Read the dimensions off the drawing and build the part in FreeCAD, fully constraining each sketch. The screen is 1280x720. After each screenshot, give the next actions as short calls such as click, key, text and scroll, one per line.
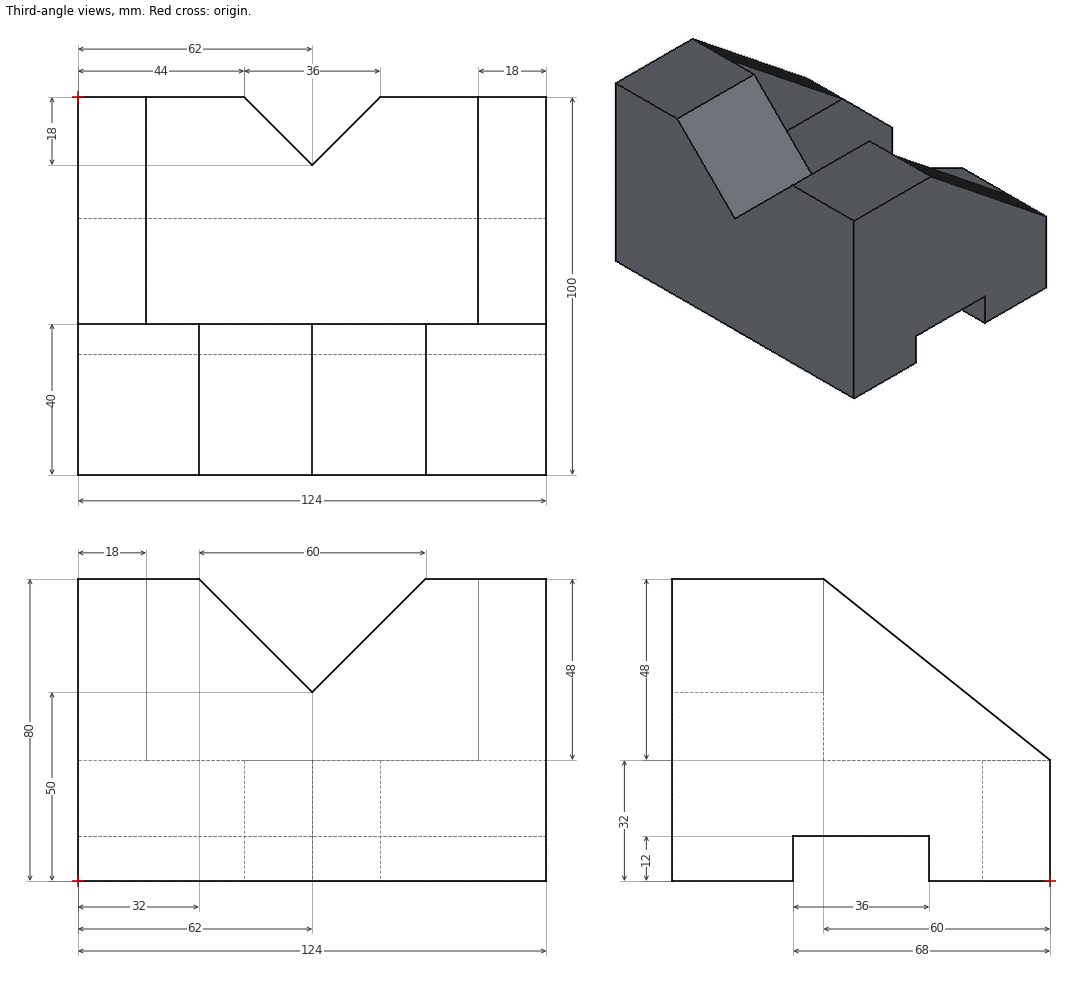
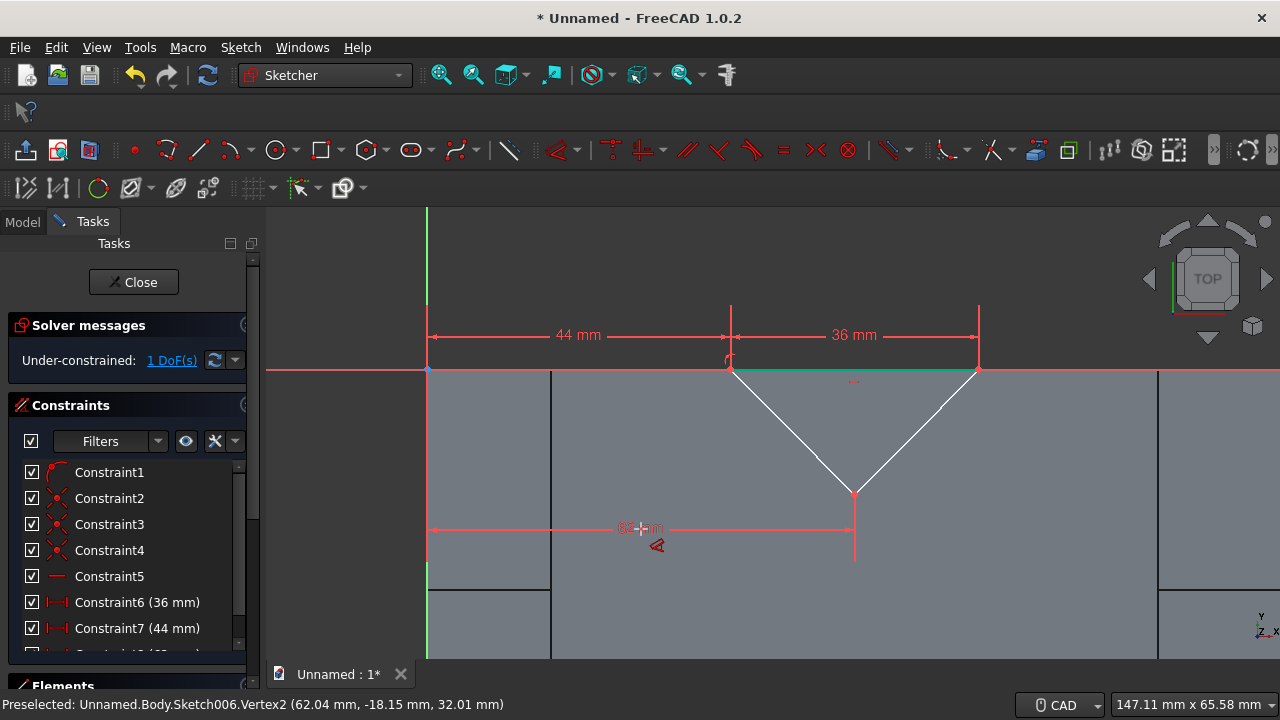
click(855, 495)
click(393, 432)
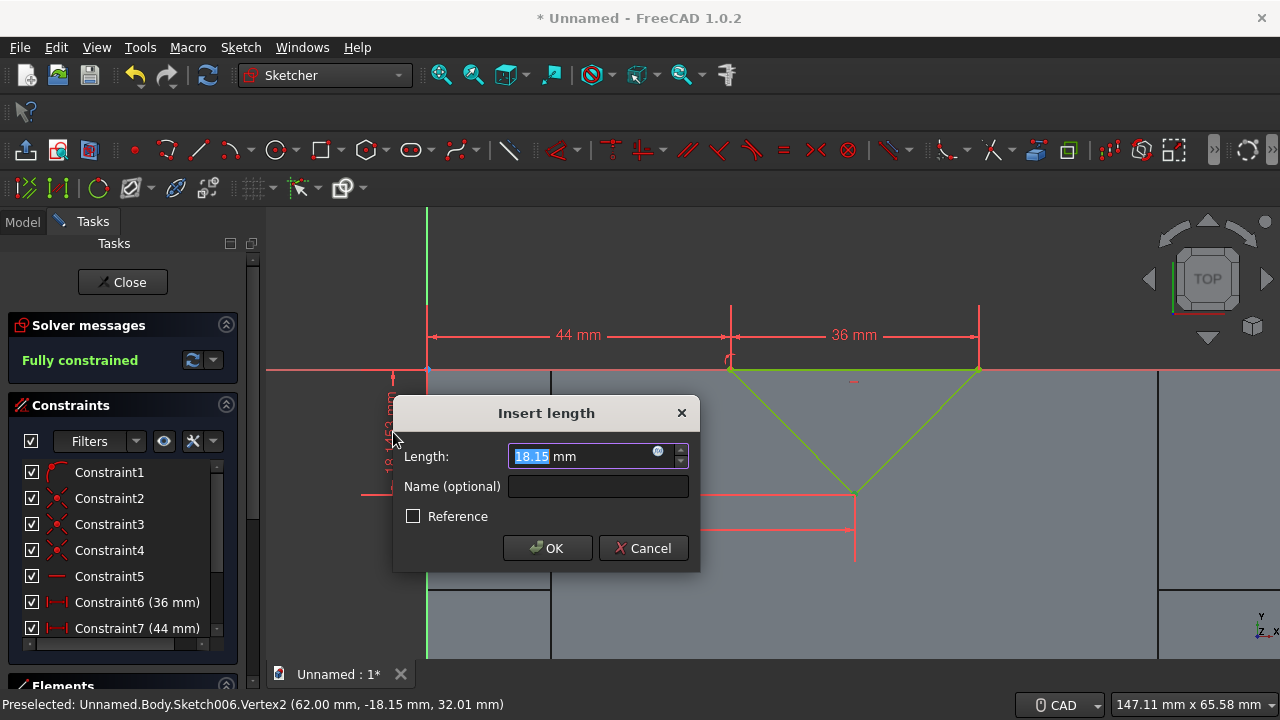
text(18)
key(Return)
key(Escape)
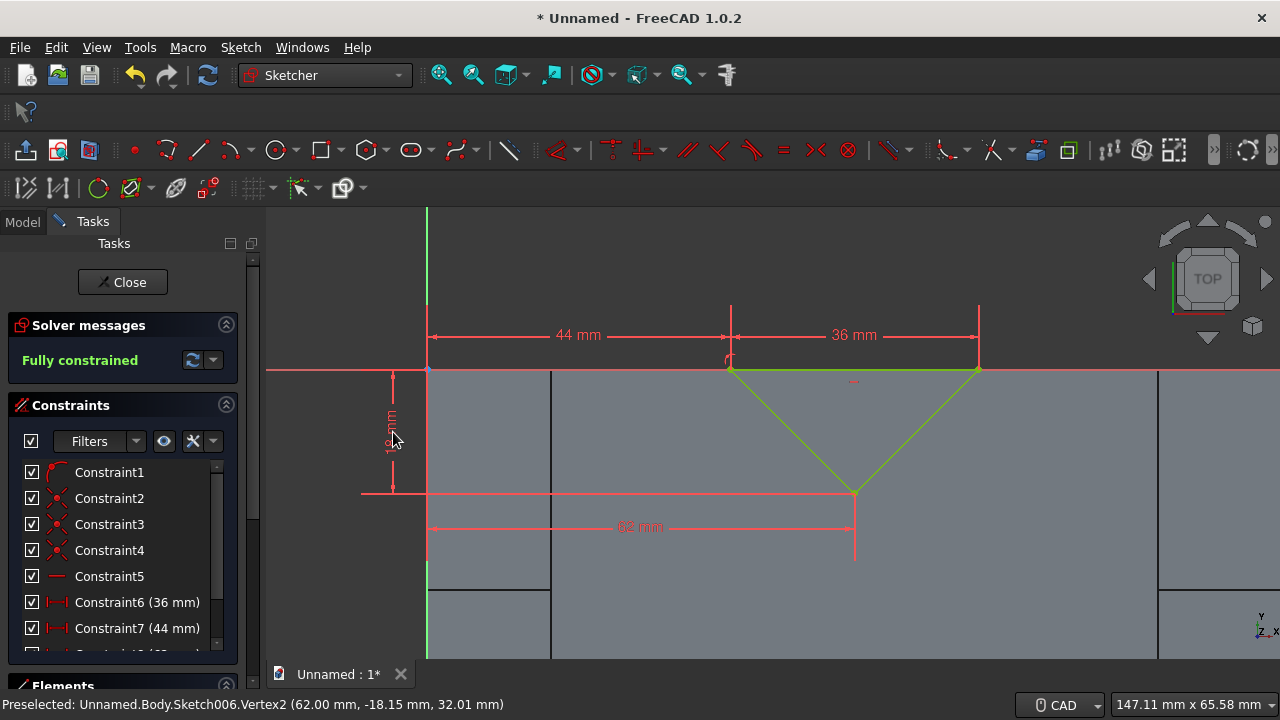
click(123, 282)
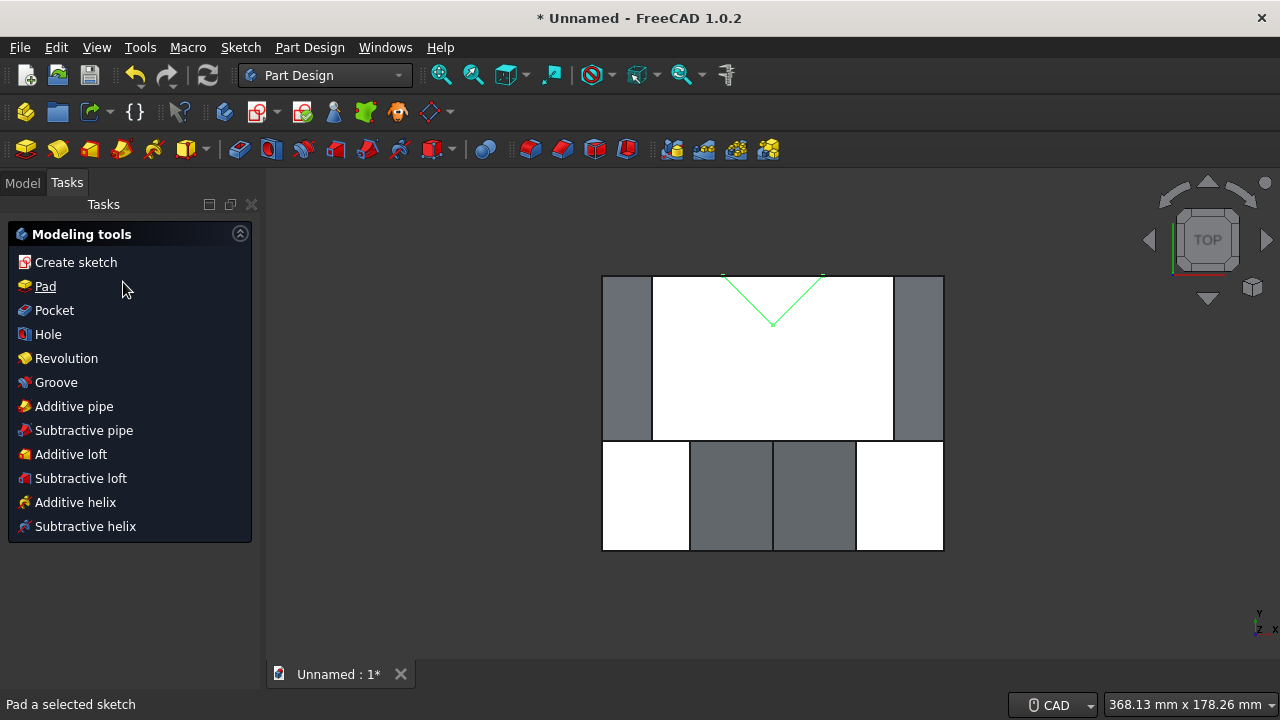
click(240, 150)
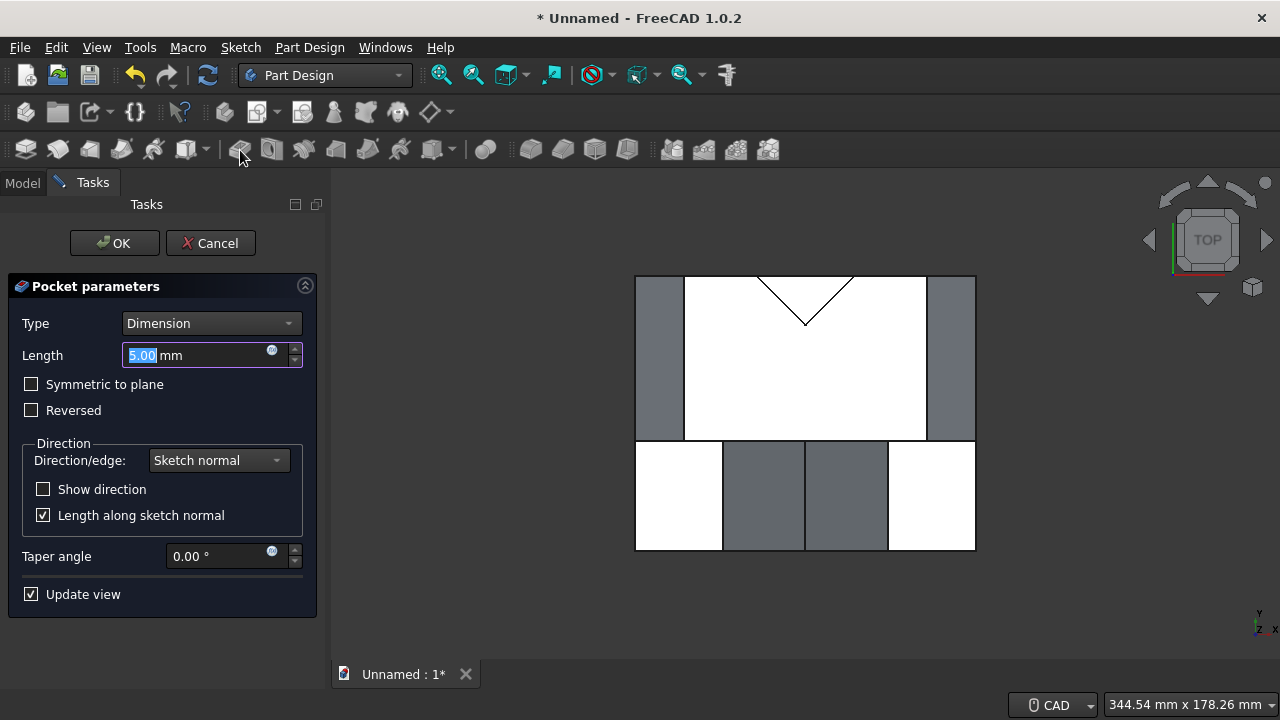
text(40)
key(Tab)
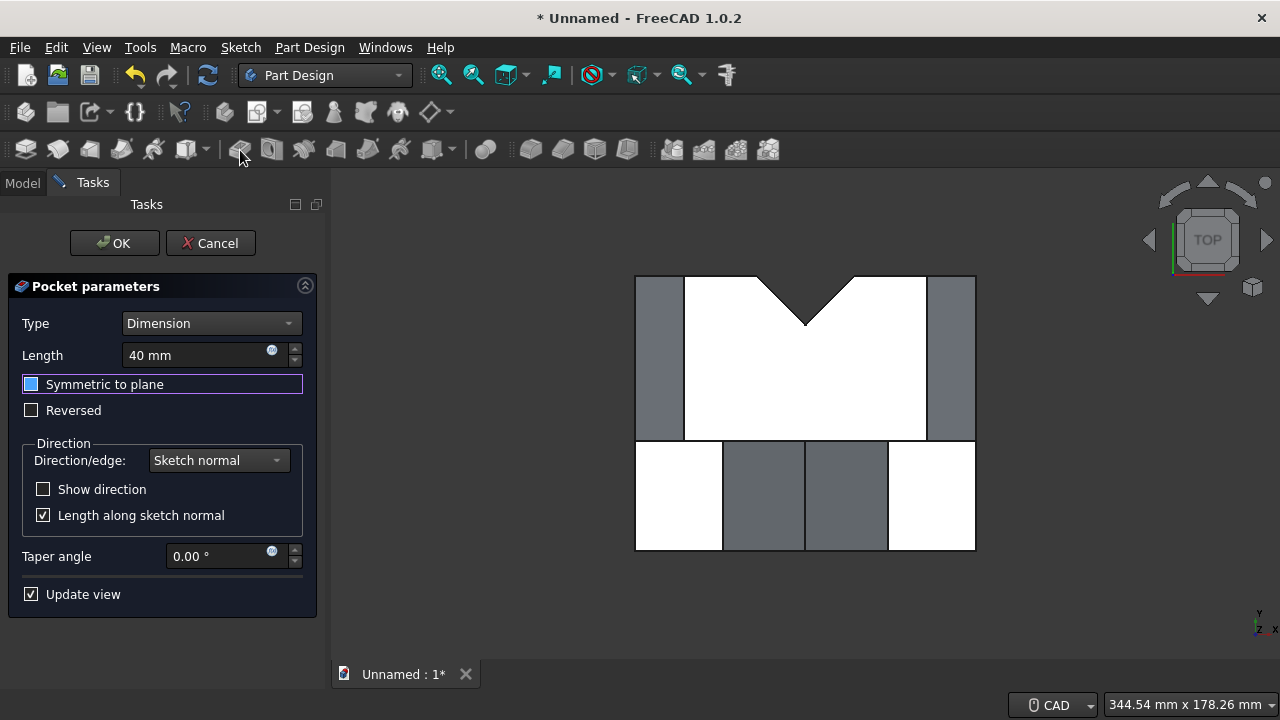
click(115, 243)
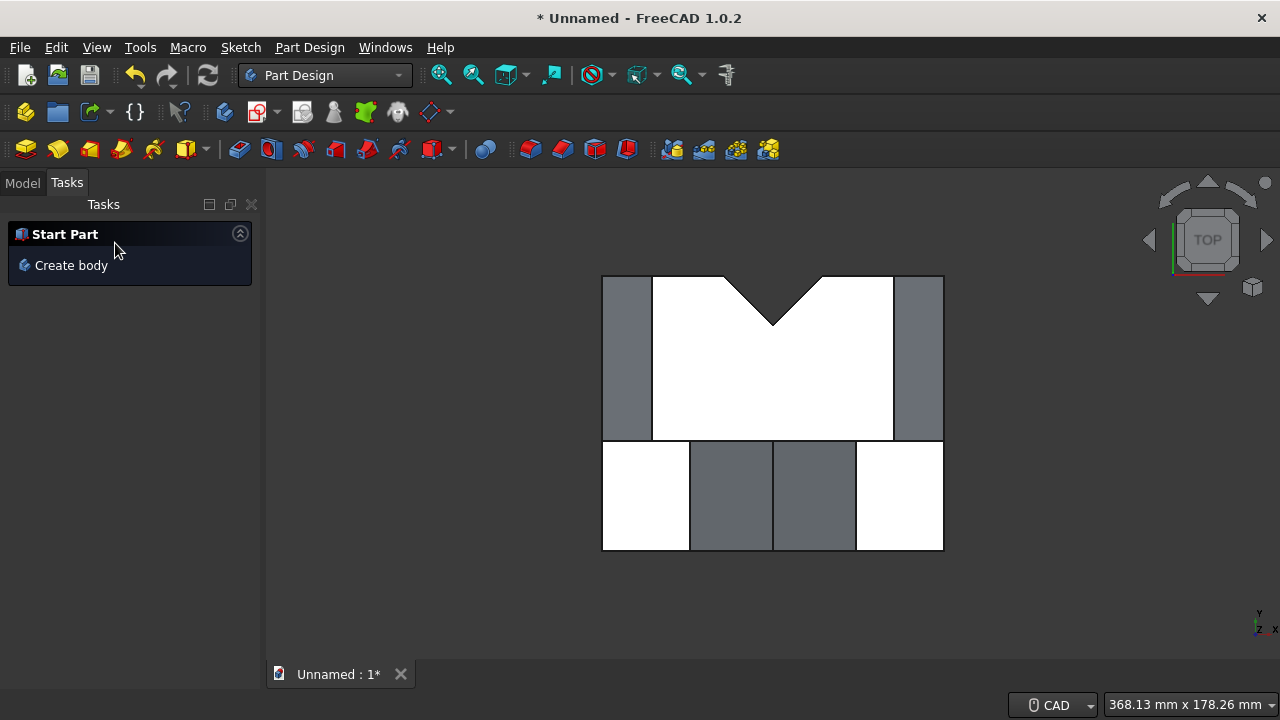
key(0)